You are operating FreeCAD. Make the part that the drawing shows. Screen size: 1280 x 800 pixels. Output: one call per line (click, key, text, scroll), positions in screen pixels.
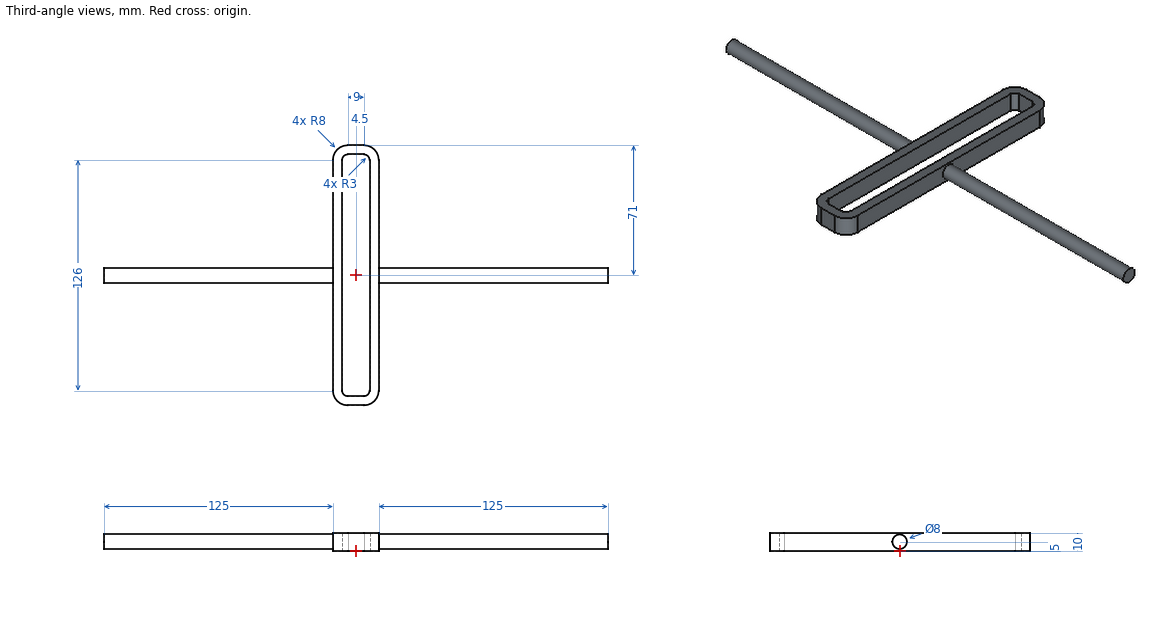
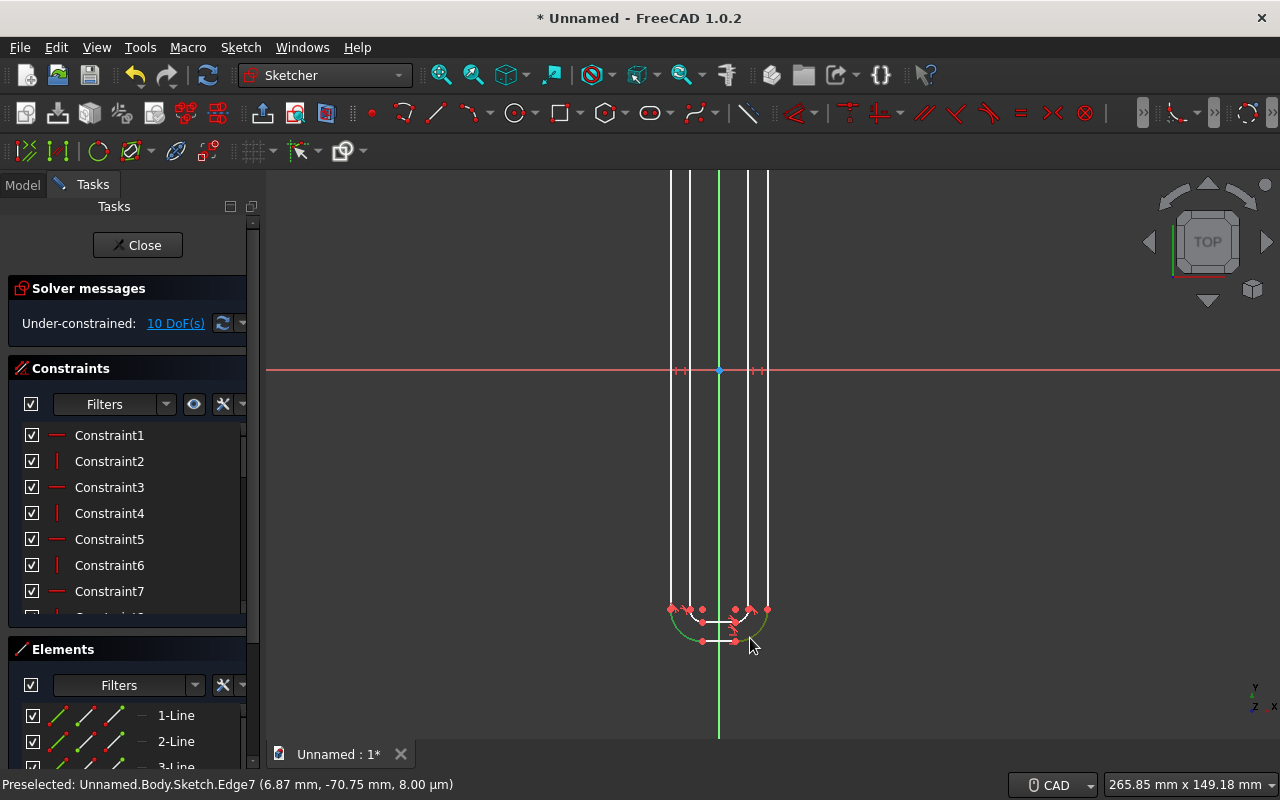
scroll(674, 626, down, 2)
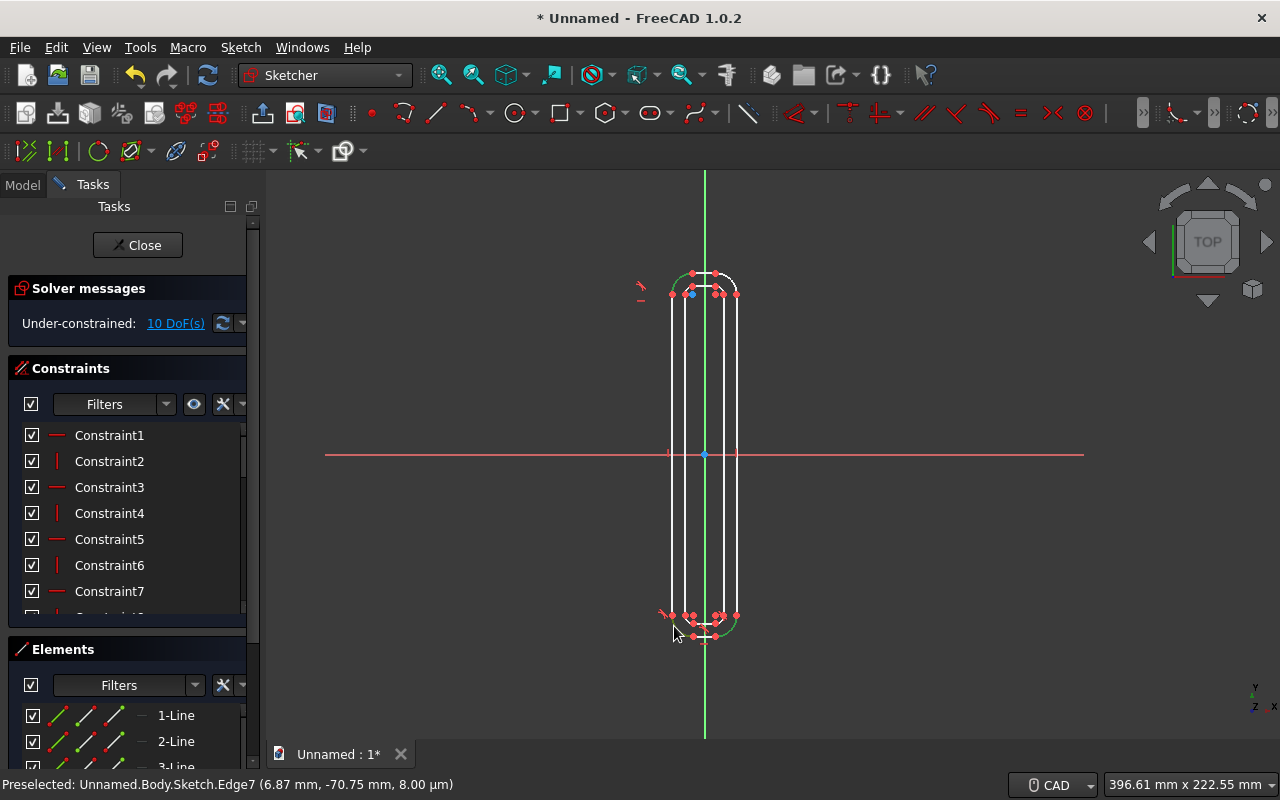
scroll(735, 285, up, 2)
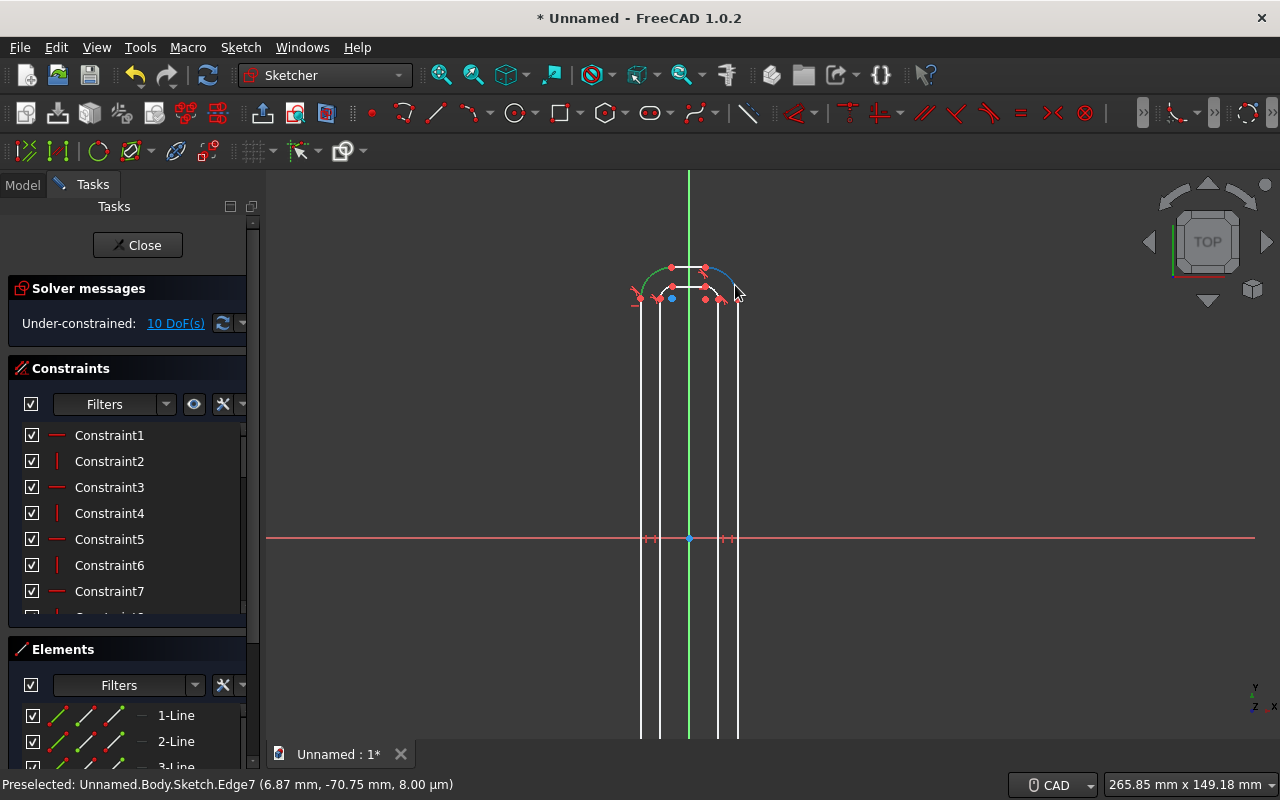
click(734, 285)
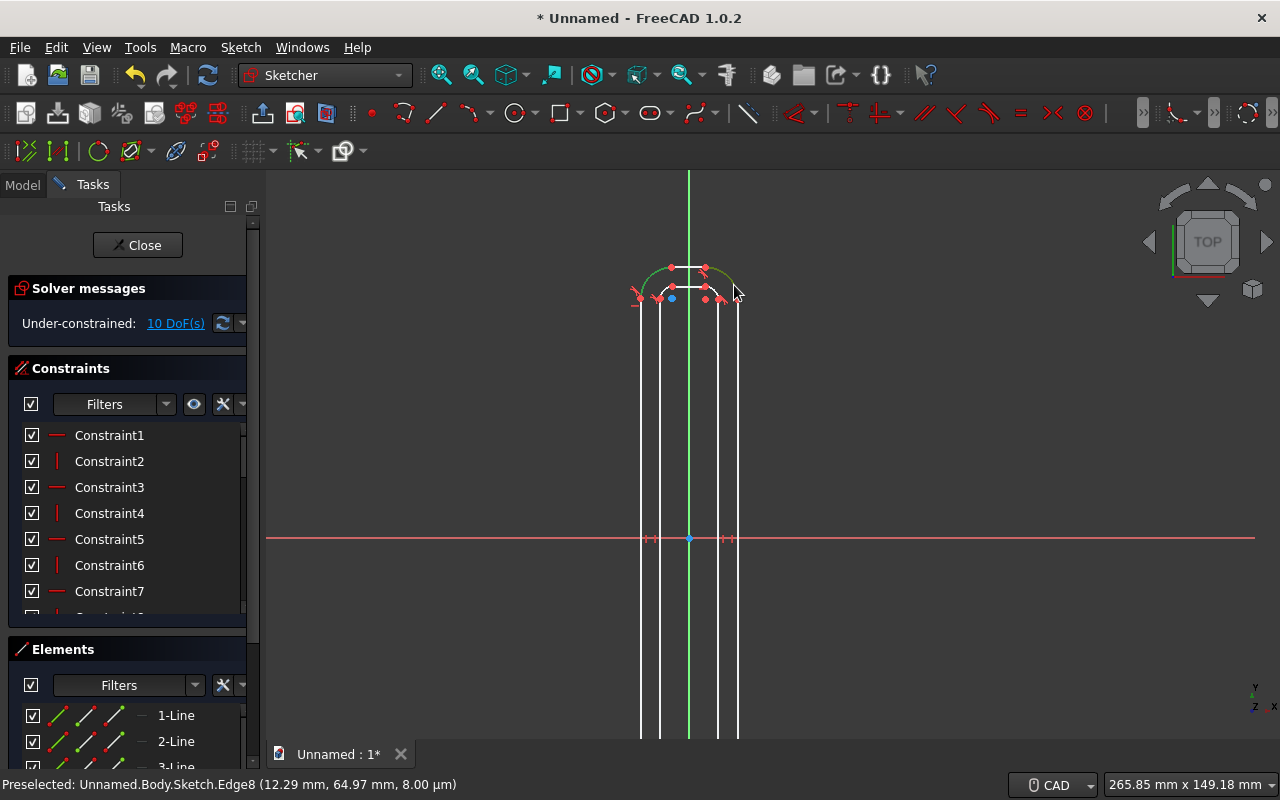
click(1022, 114)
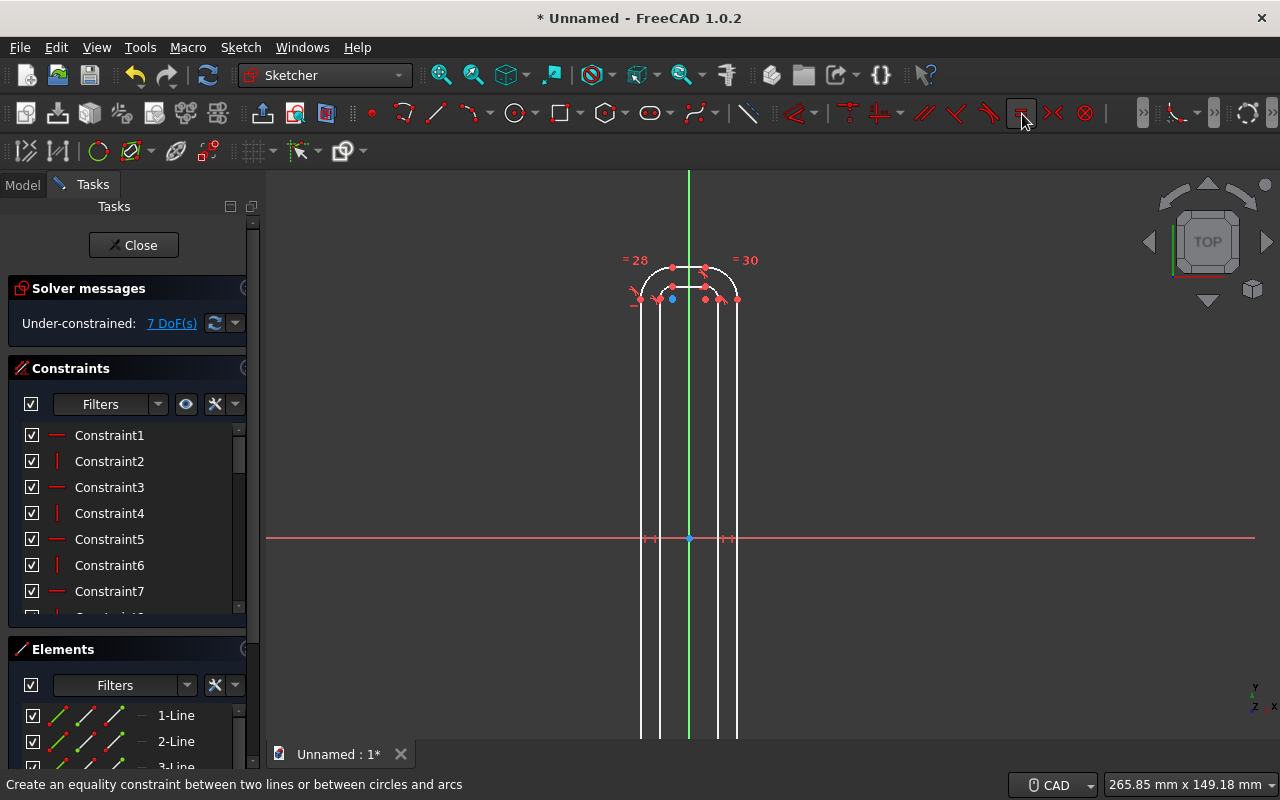
scroll(715, 290, up, 2)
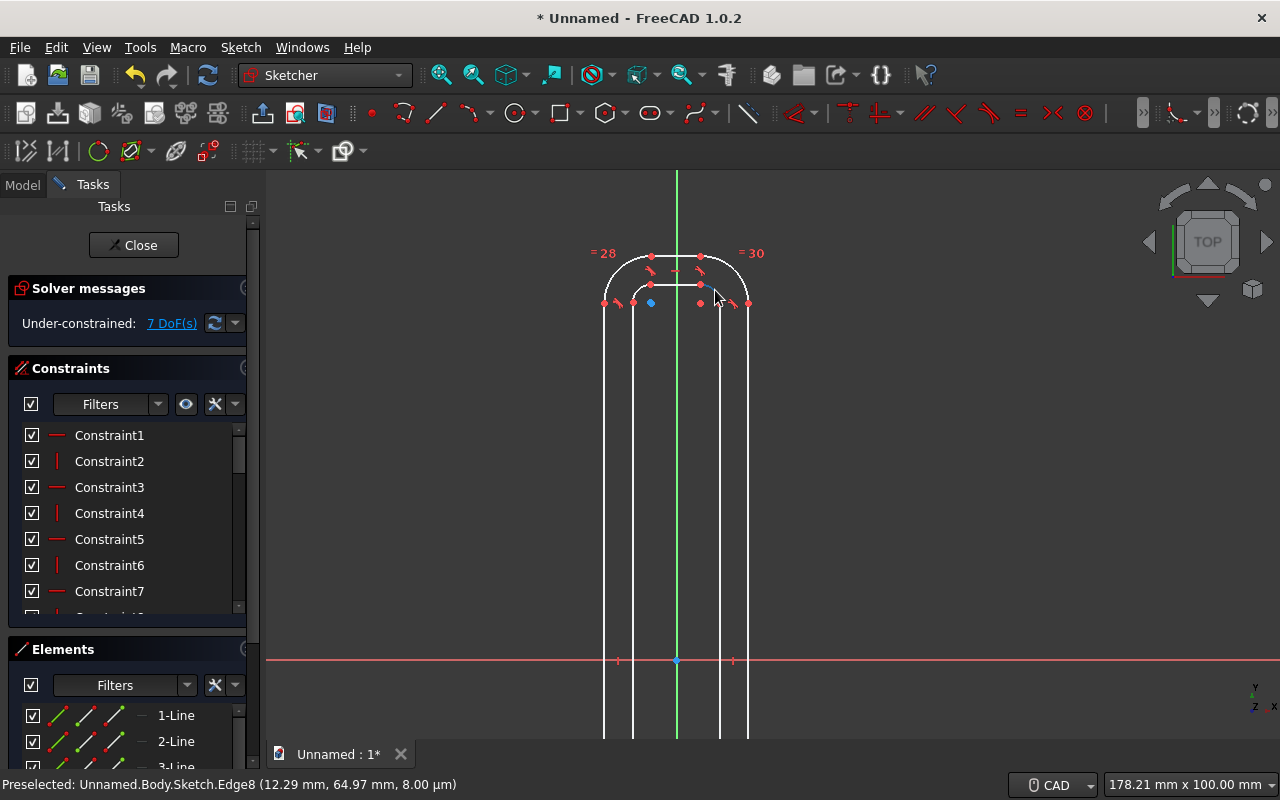
click(714, 290)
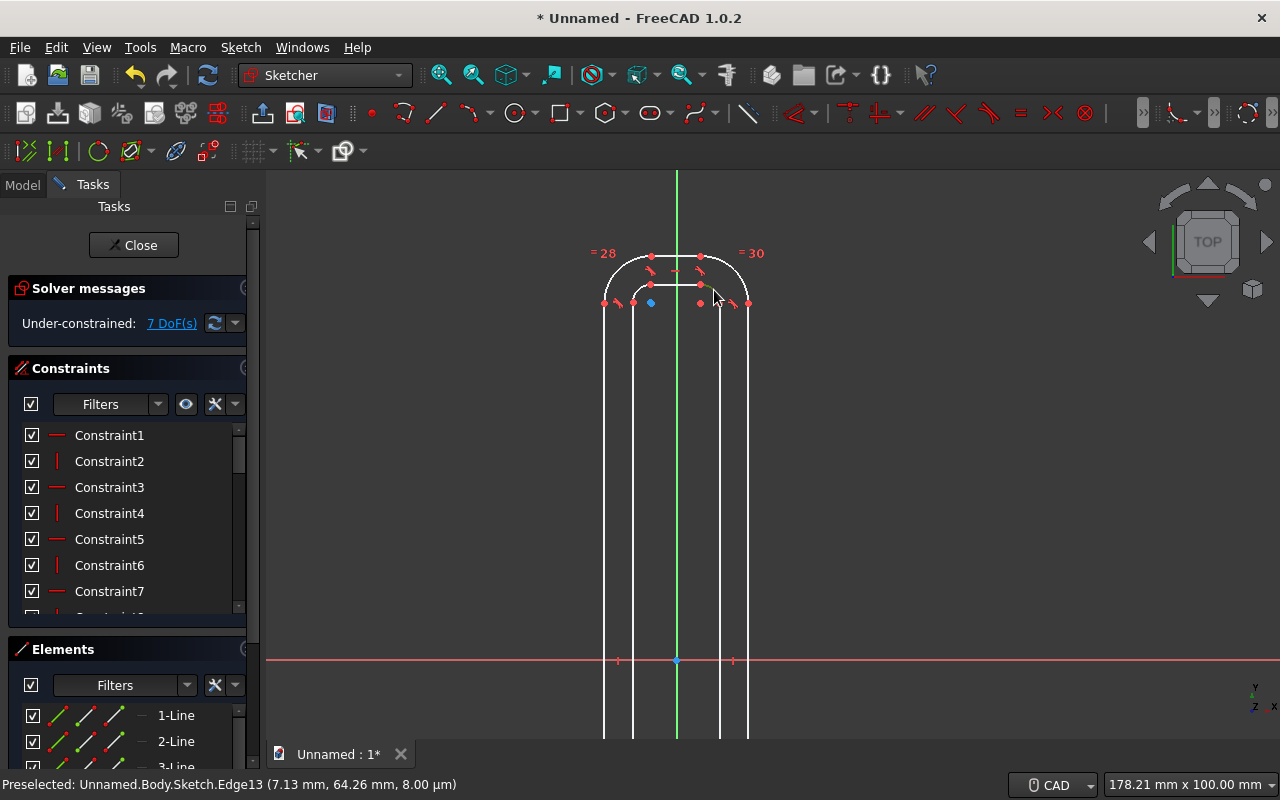
click(638, 290)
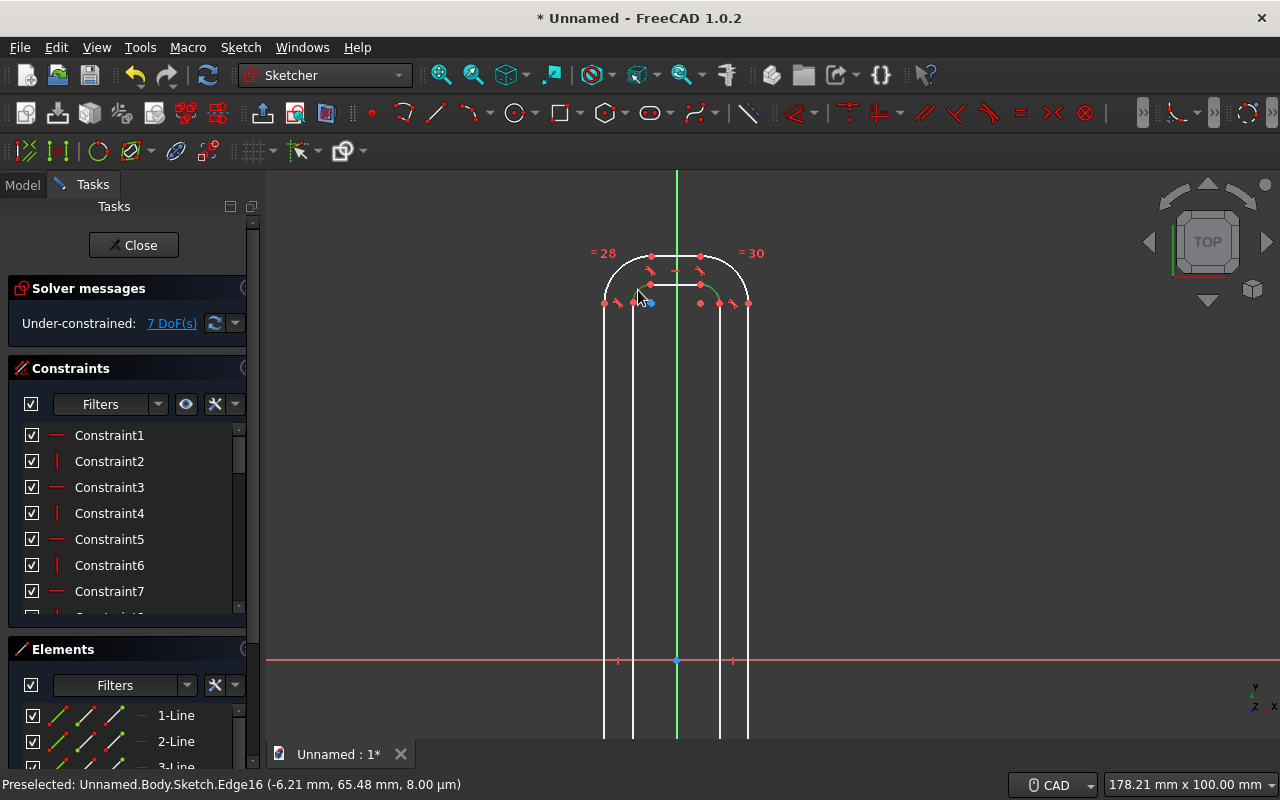
click(1022, 114)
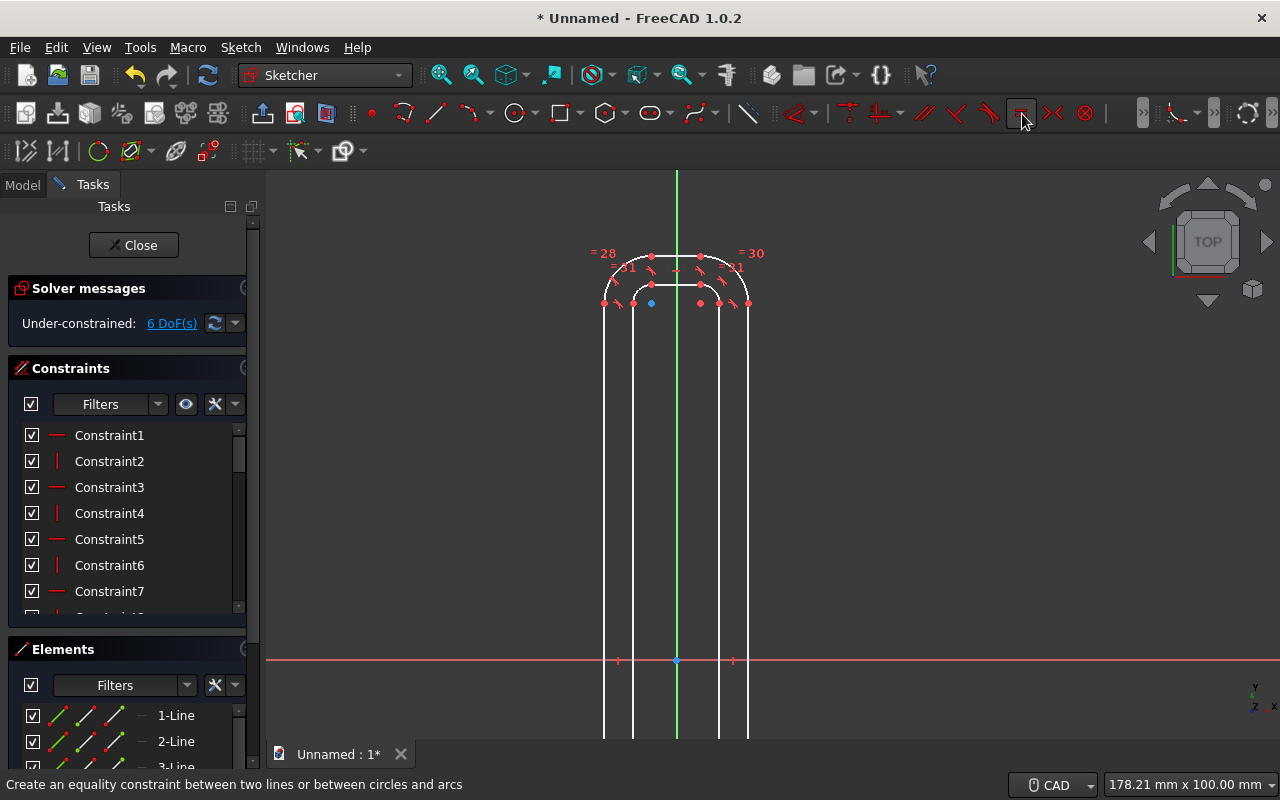
click(637, 258)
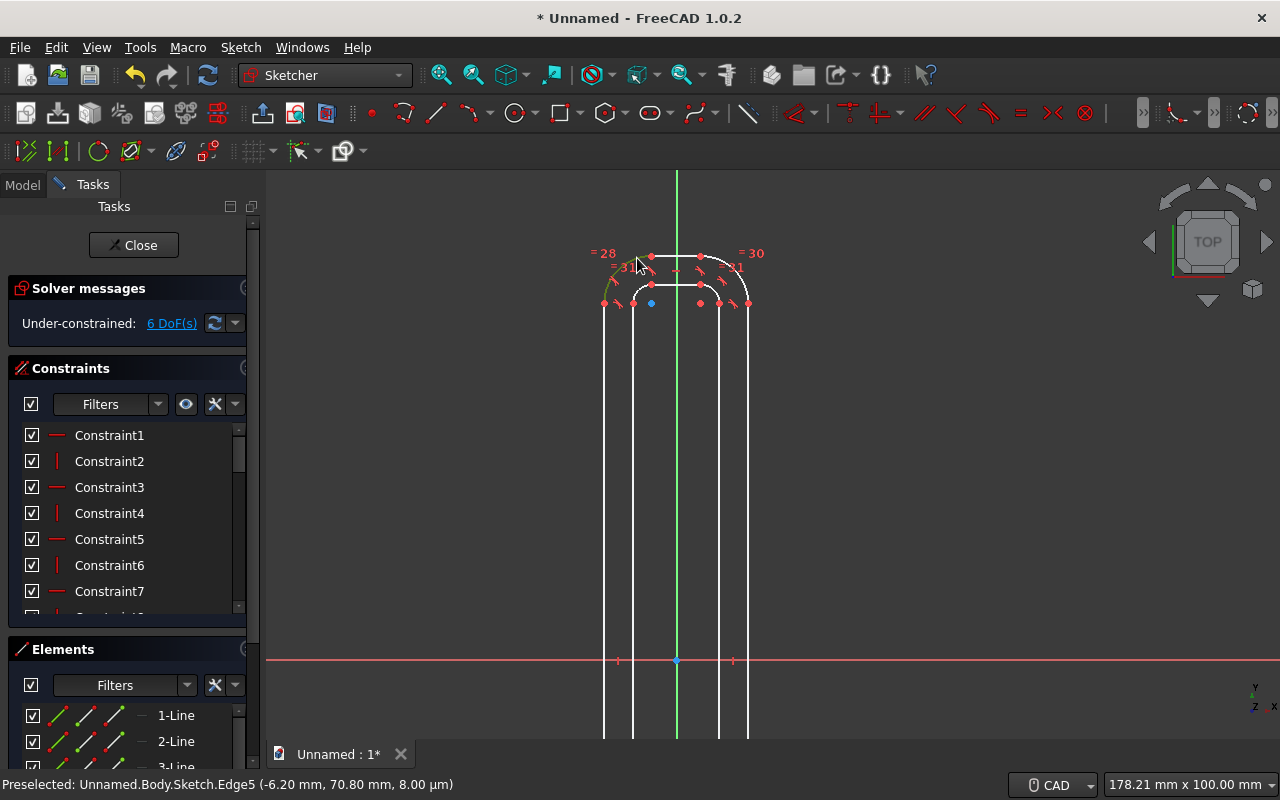
click(816, 114)